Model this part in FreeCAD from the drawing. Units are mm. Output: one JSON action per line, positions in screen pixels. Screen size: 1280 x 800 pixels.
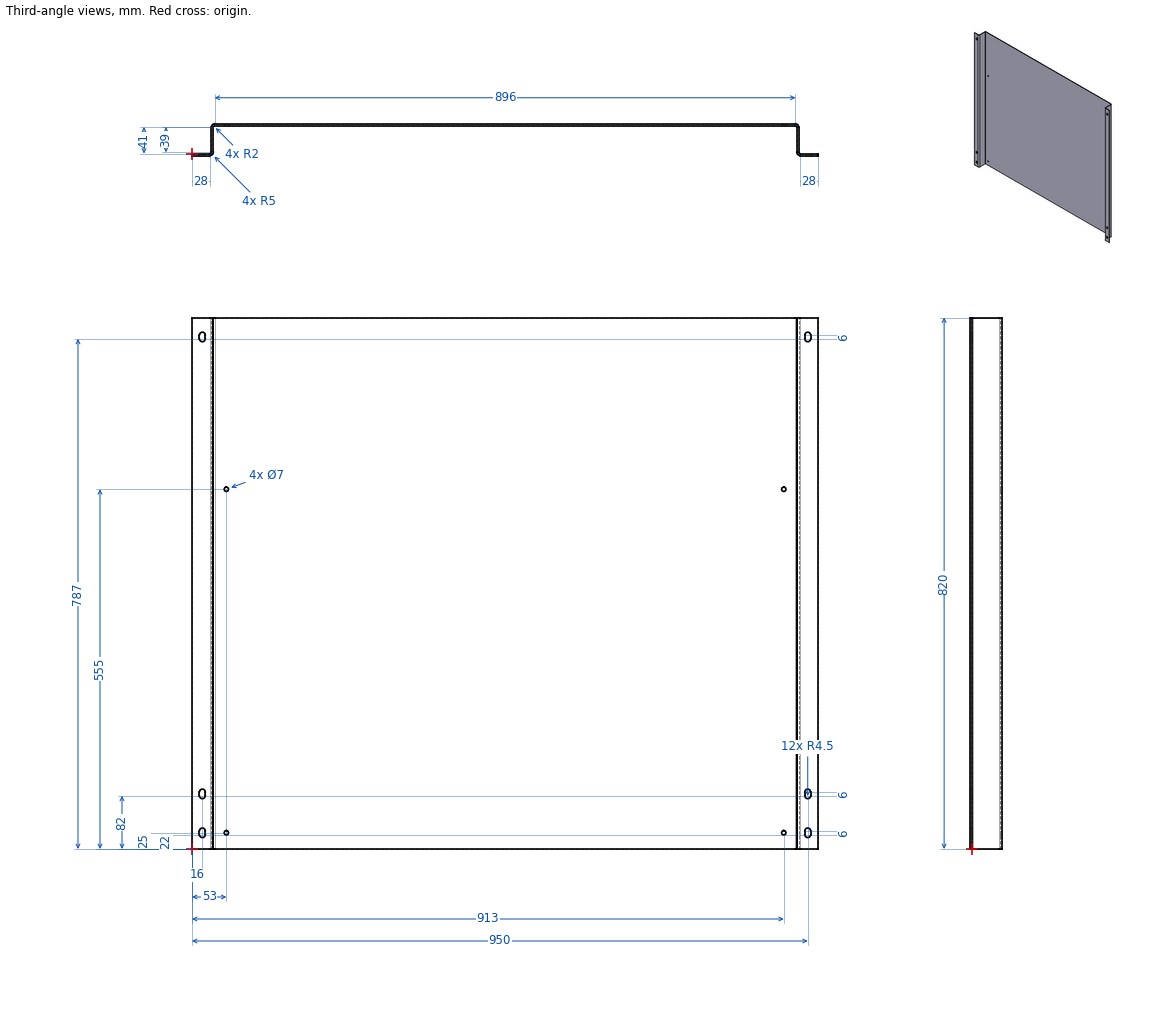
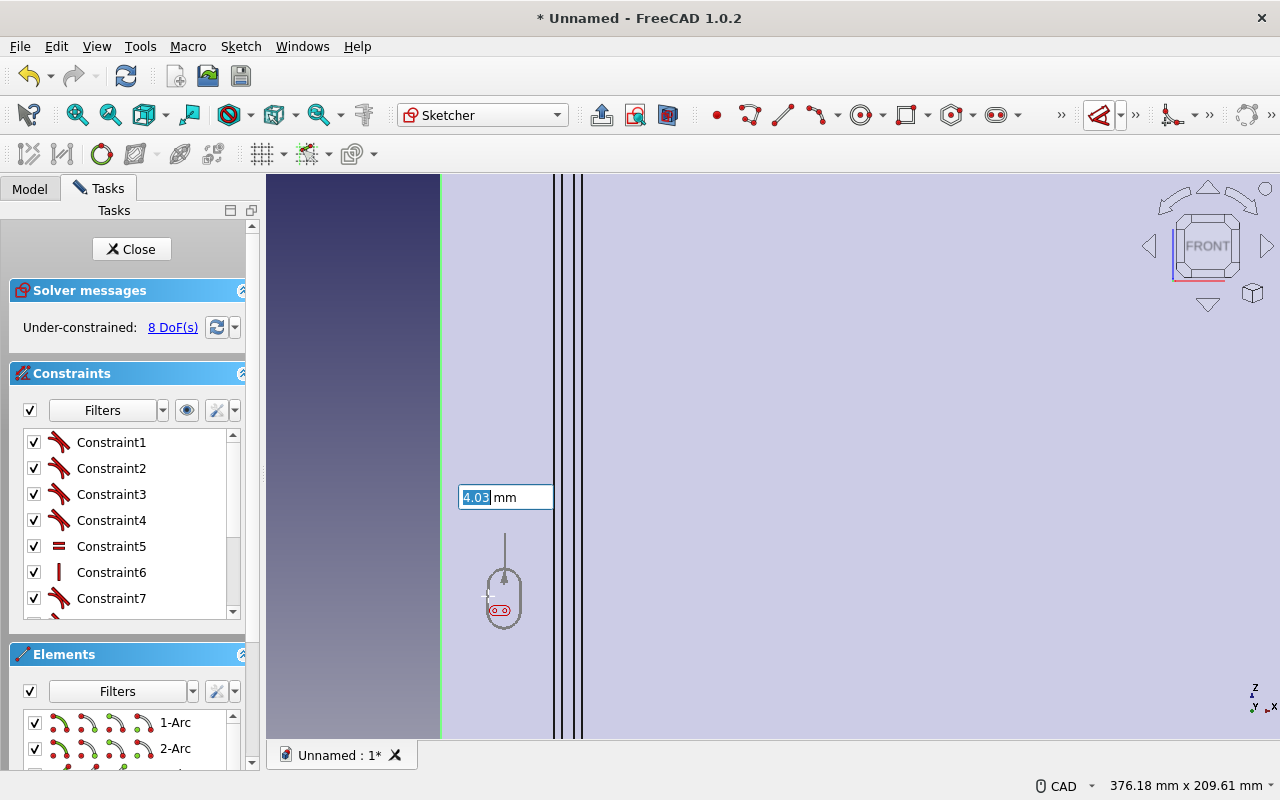
{"action": "left_click", "coordinate": [487, 596]}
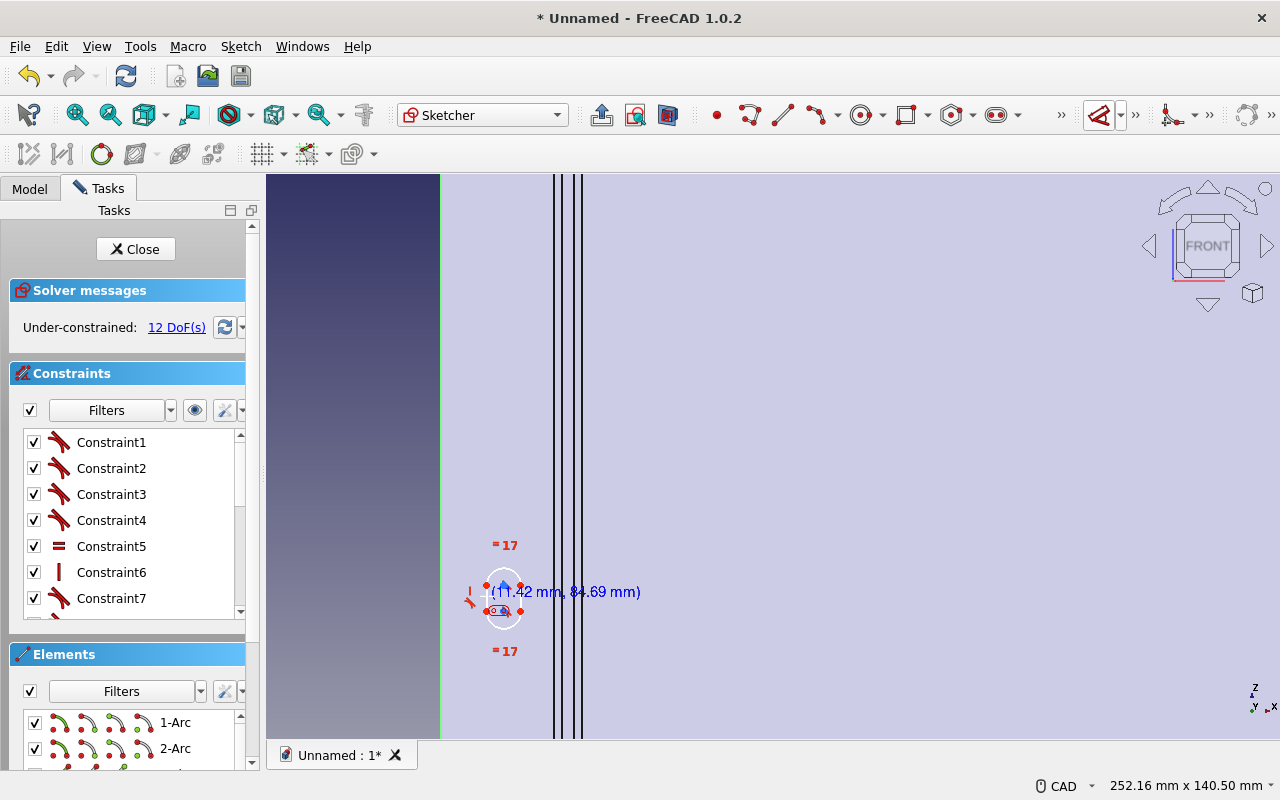
{"action": "scroll", "coordinate": [498, 596], "scroll_direction": "down", "scroll_amount": 11}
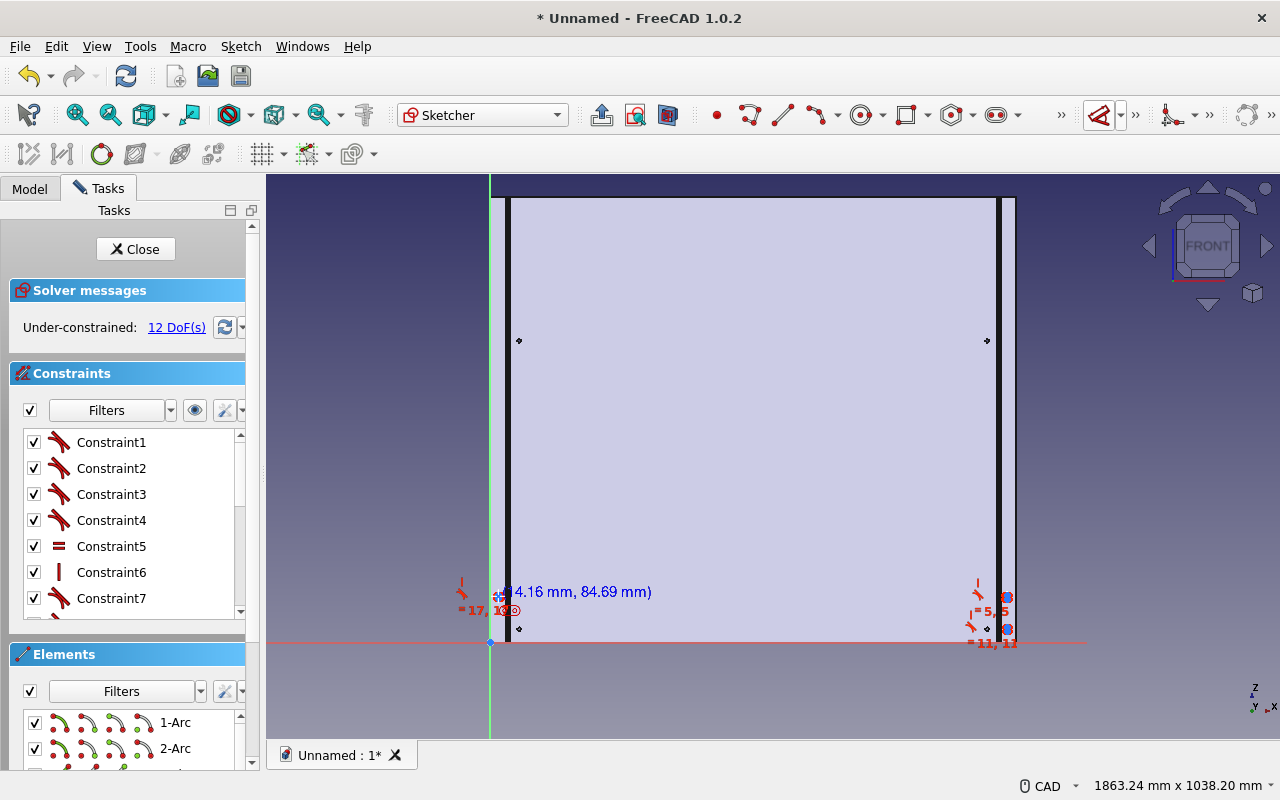
{"action": "scroll", "coordinate": [499, 625], "scroll_direction": "up", "scroll_amount": 13}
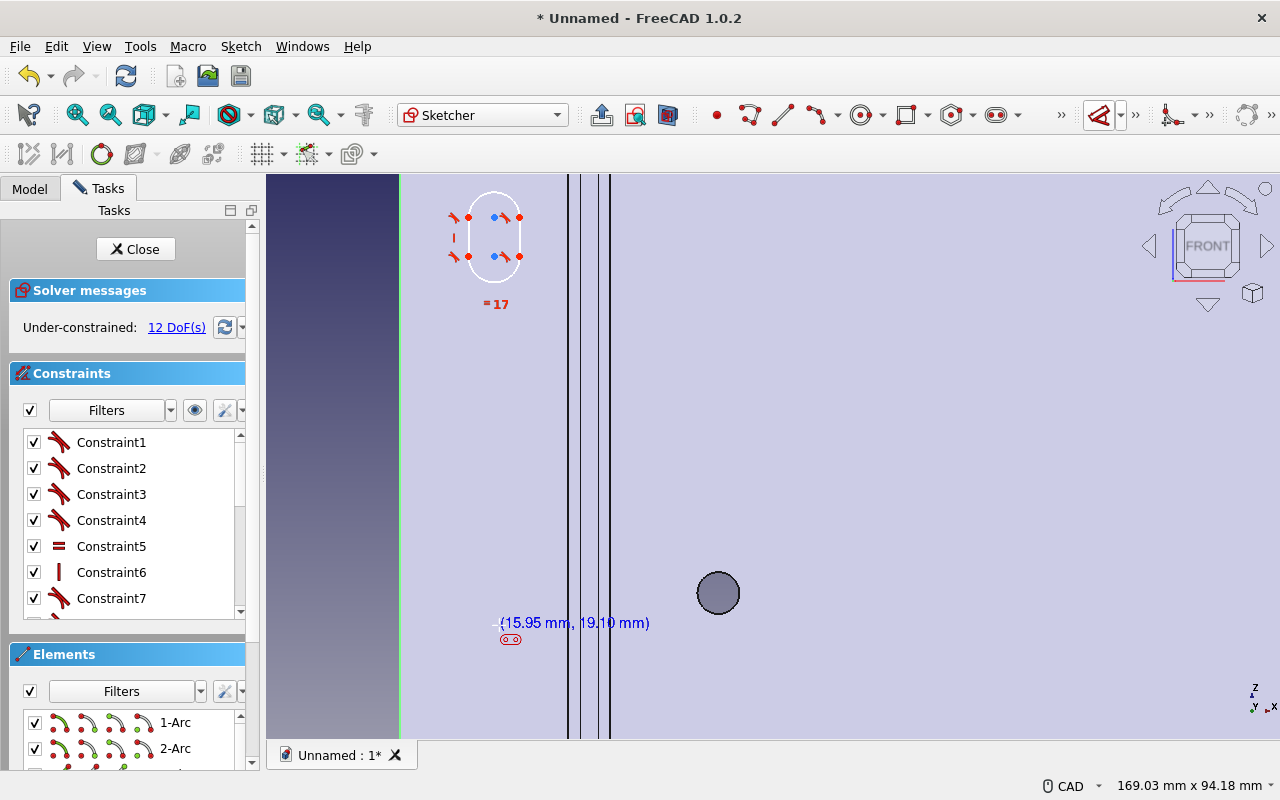
{"action": "scroll", "coordinate": [499, 625], "scroll_direction": "down", "scroll_amount": 13}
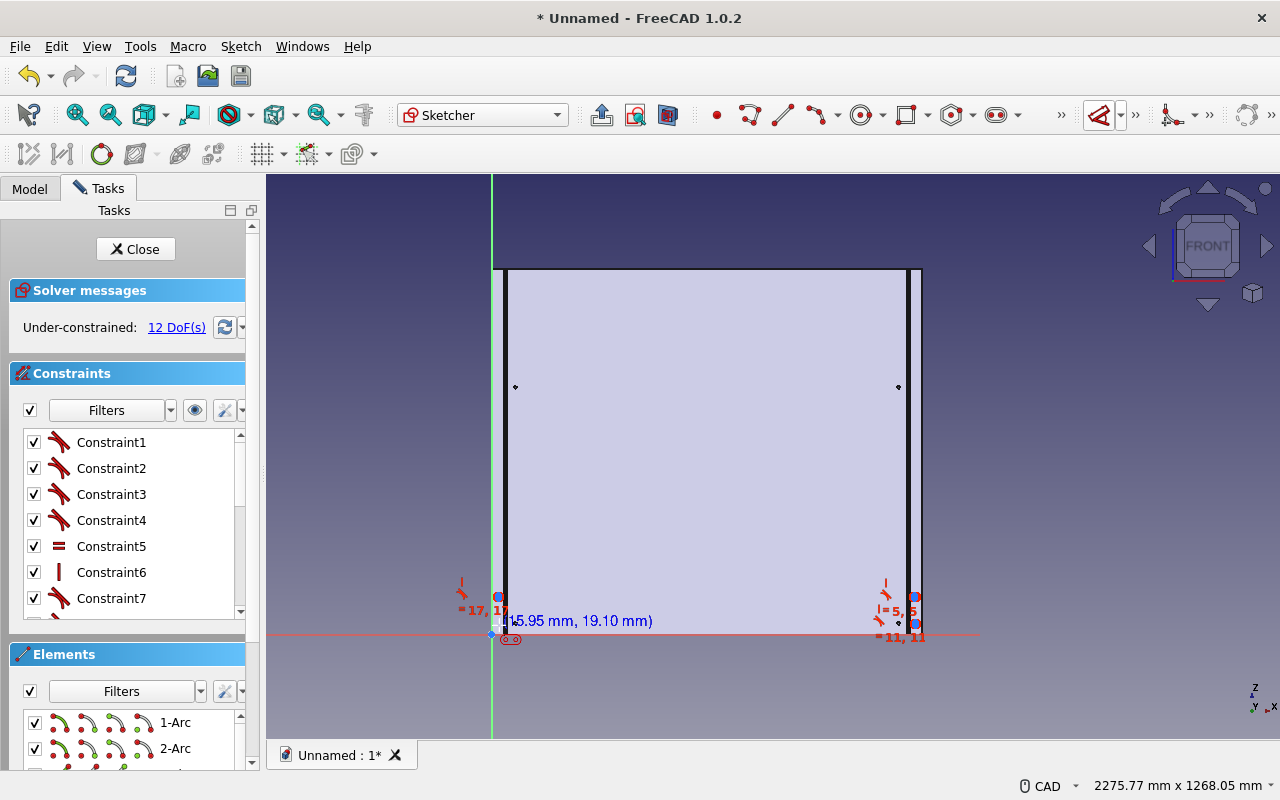
{"action": "scroll", "coordinate": [499, 625], "scroll_direction": "up", "scroll_amount": 5}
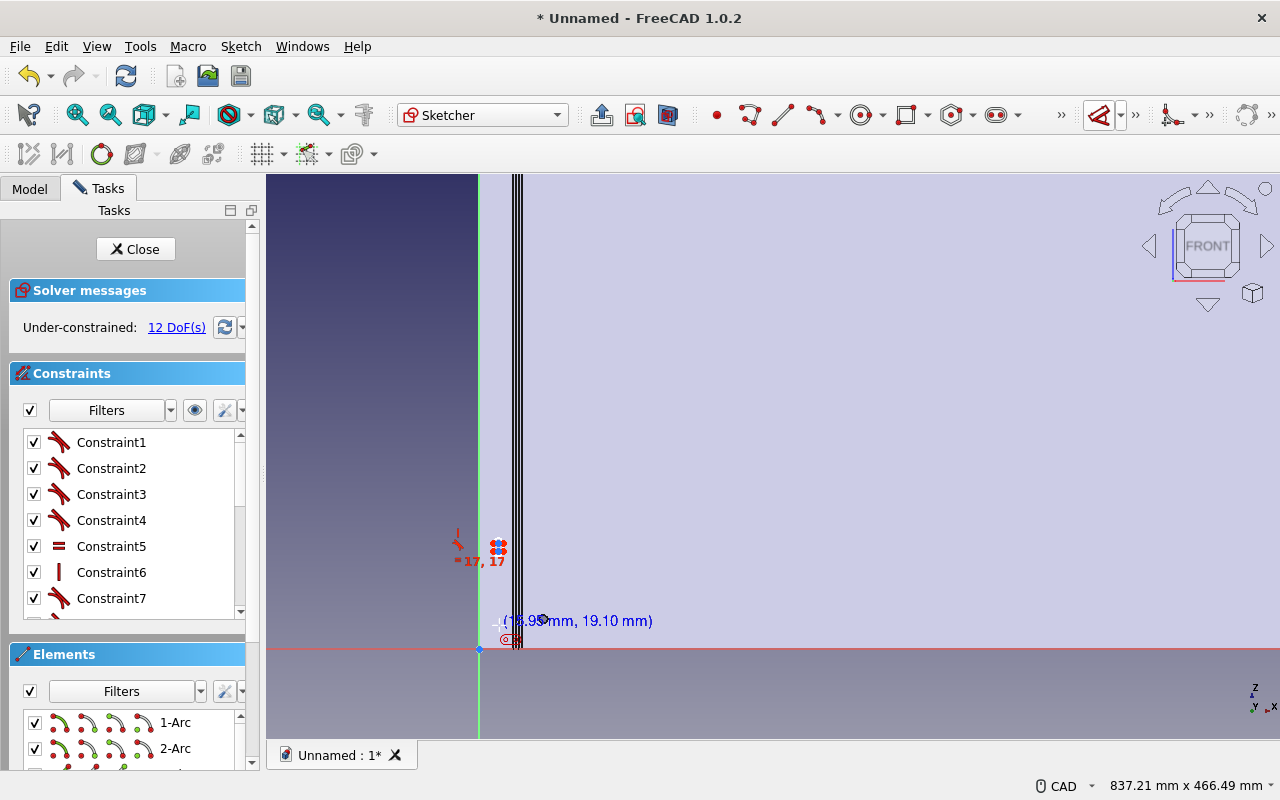
{"action": "left_click", "coordinate": [499, 623]}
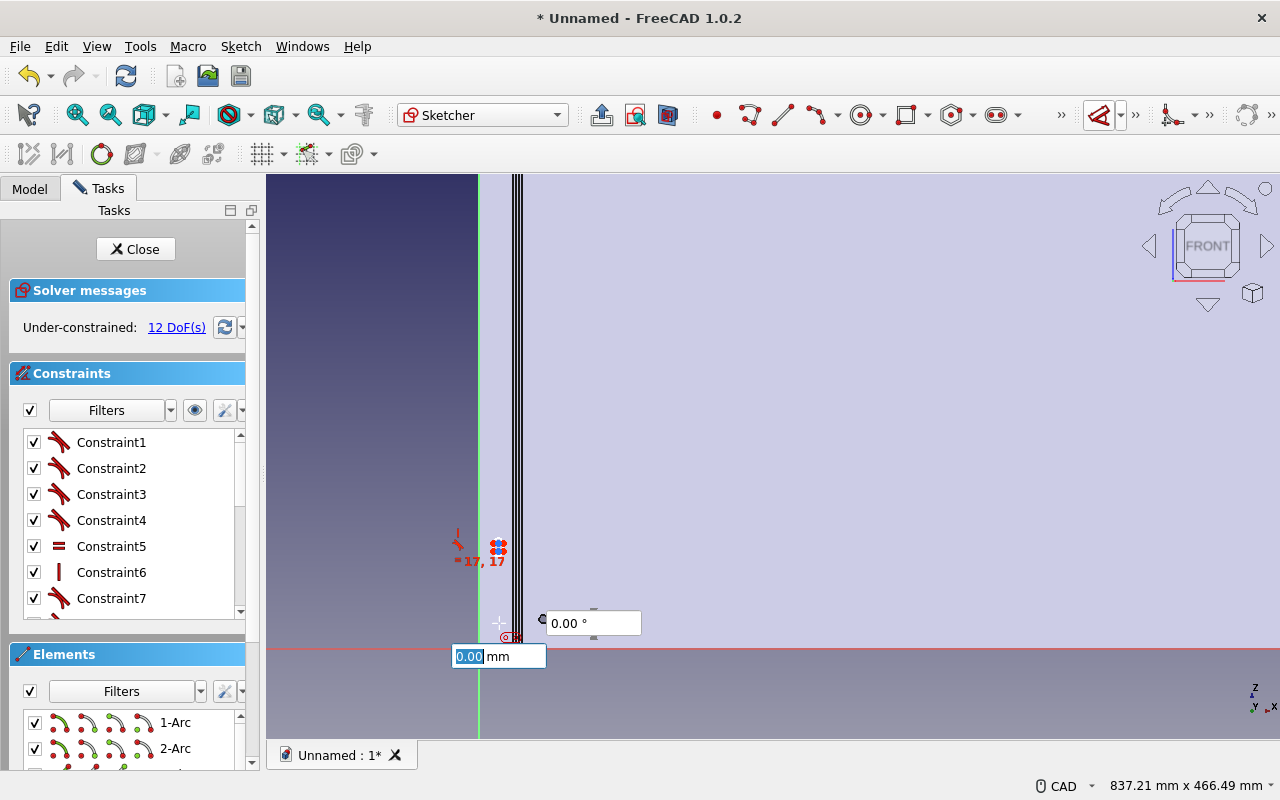
{"action": "scroll", "coordinate": [499, 616], "scroll_direction": "up", "scroll_amount": 4}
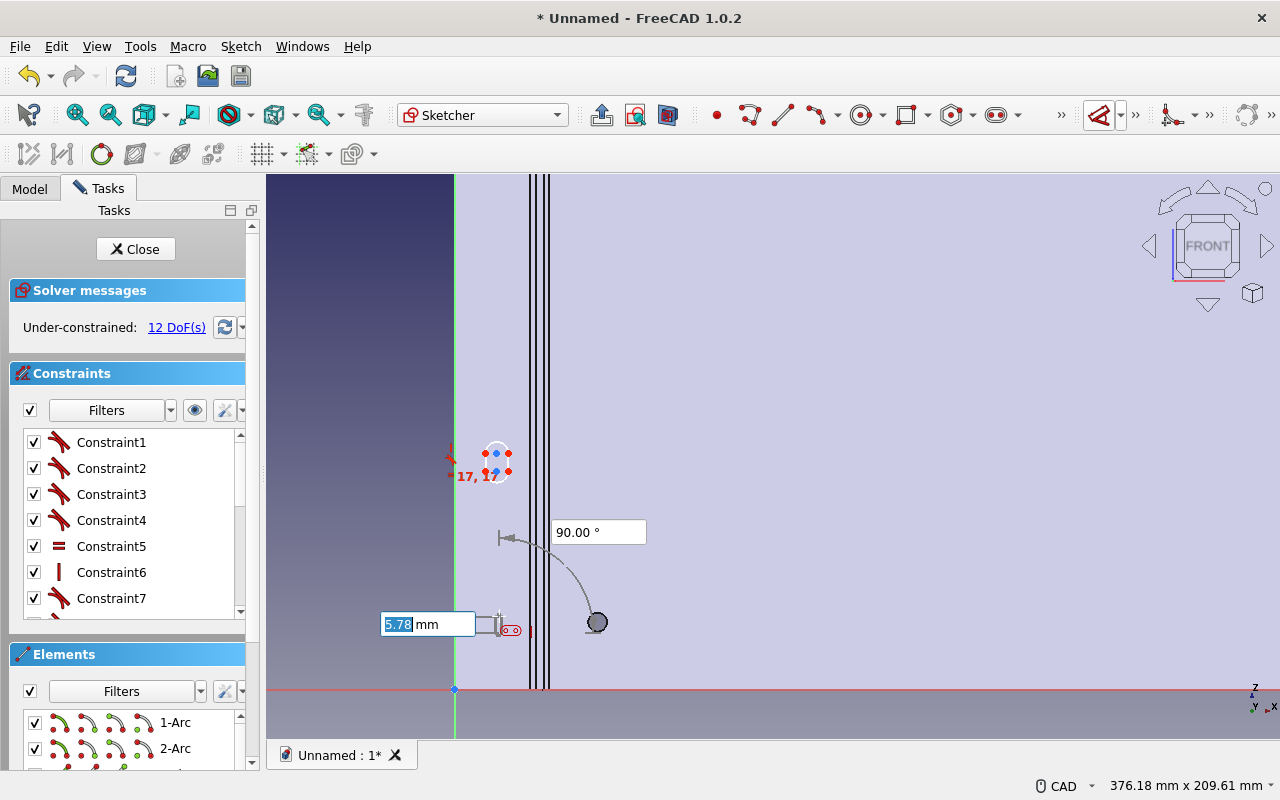
{"action": "left_click", "coordinate": [499, 614]}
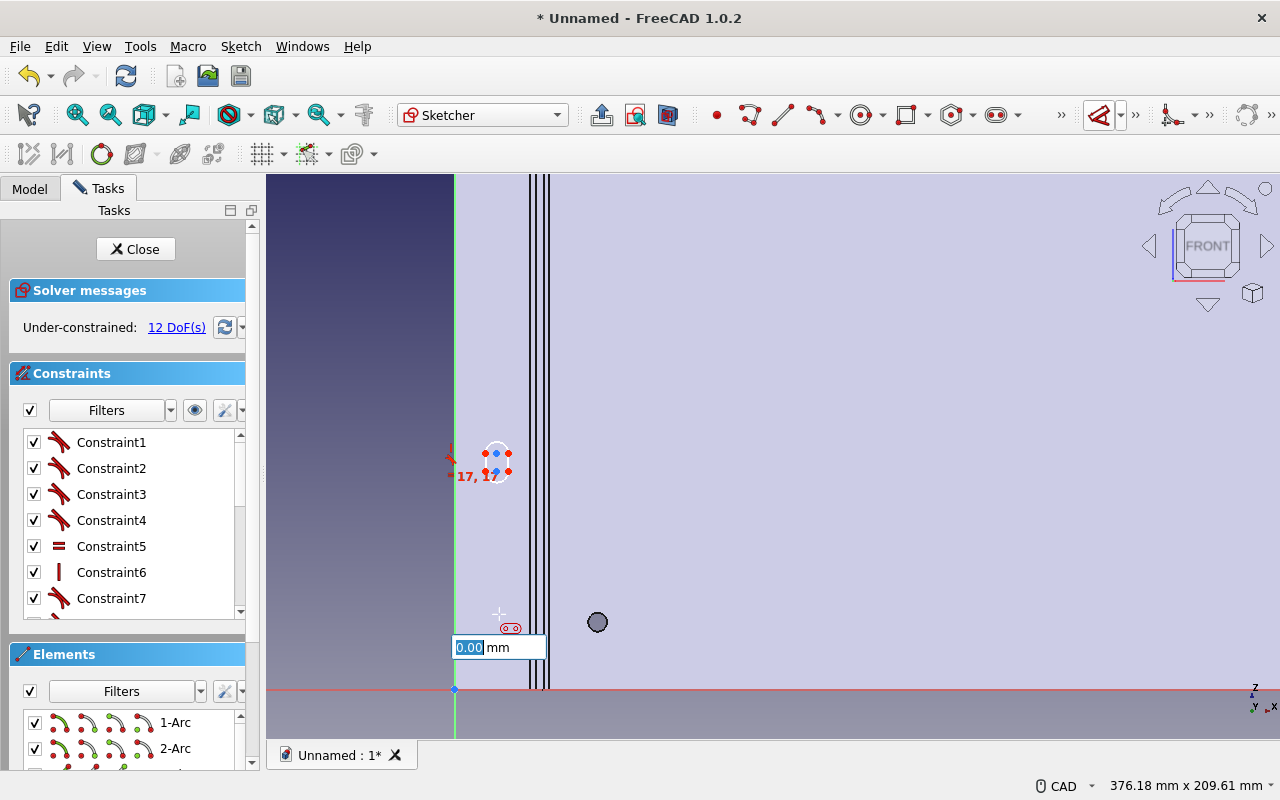
{"action": "scroll", "coordinate": [486, 622], "scroll_direction": "up", "scroll_amount": 2}